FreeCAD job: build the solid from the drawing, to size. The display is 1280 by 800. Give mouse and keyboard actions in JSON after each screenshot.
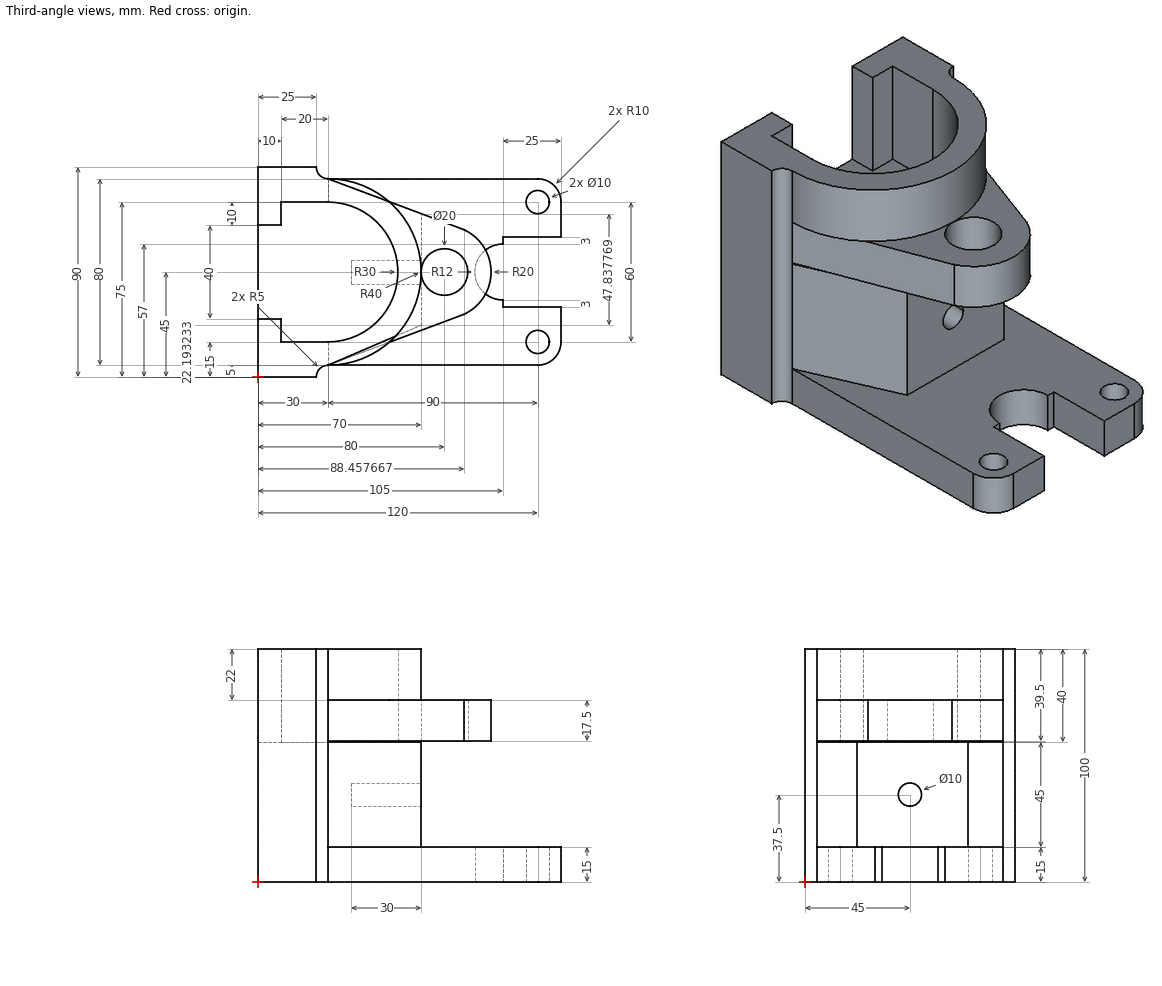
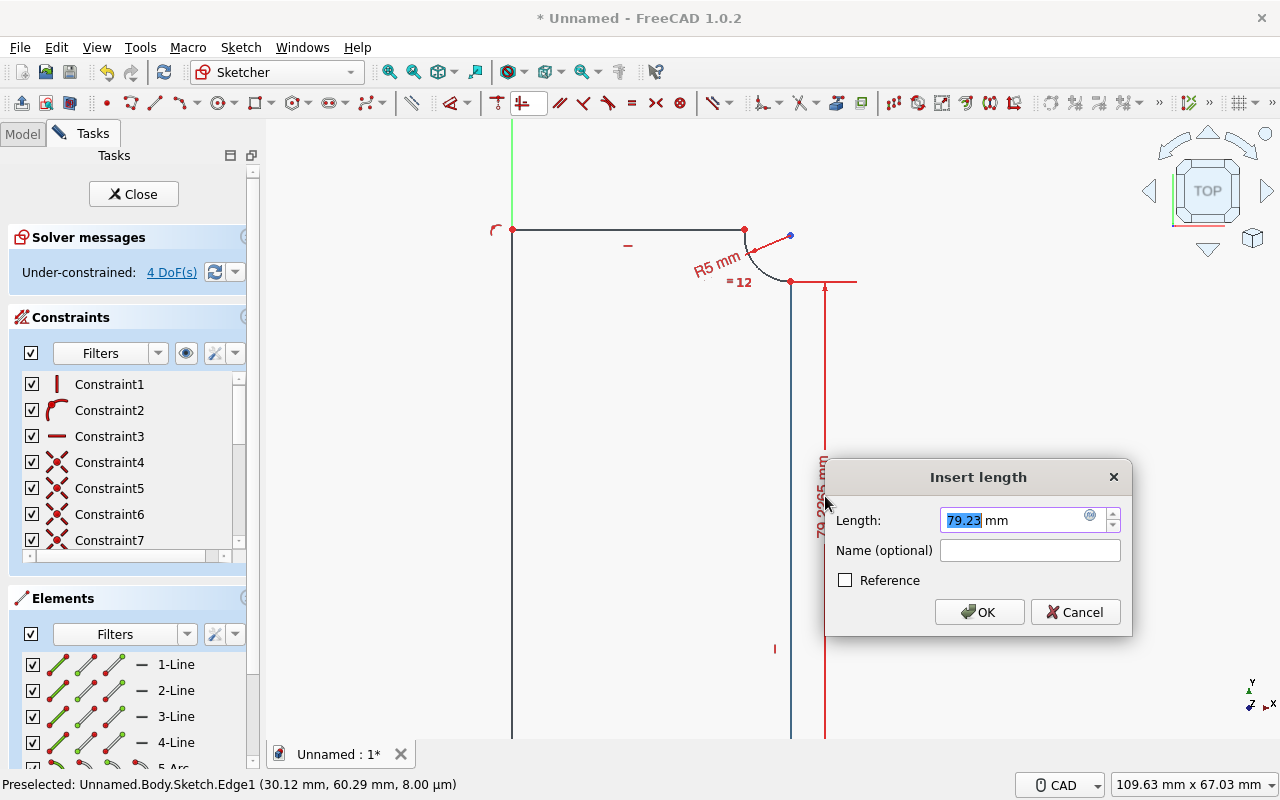
{"action": "type", "text": "80"}
{"action": "key", "text": "Return"}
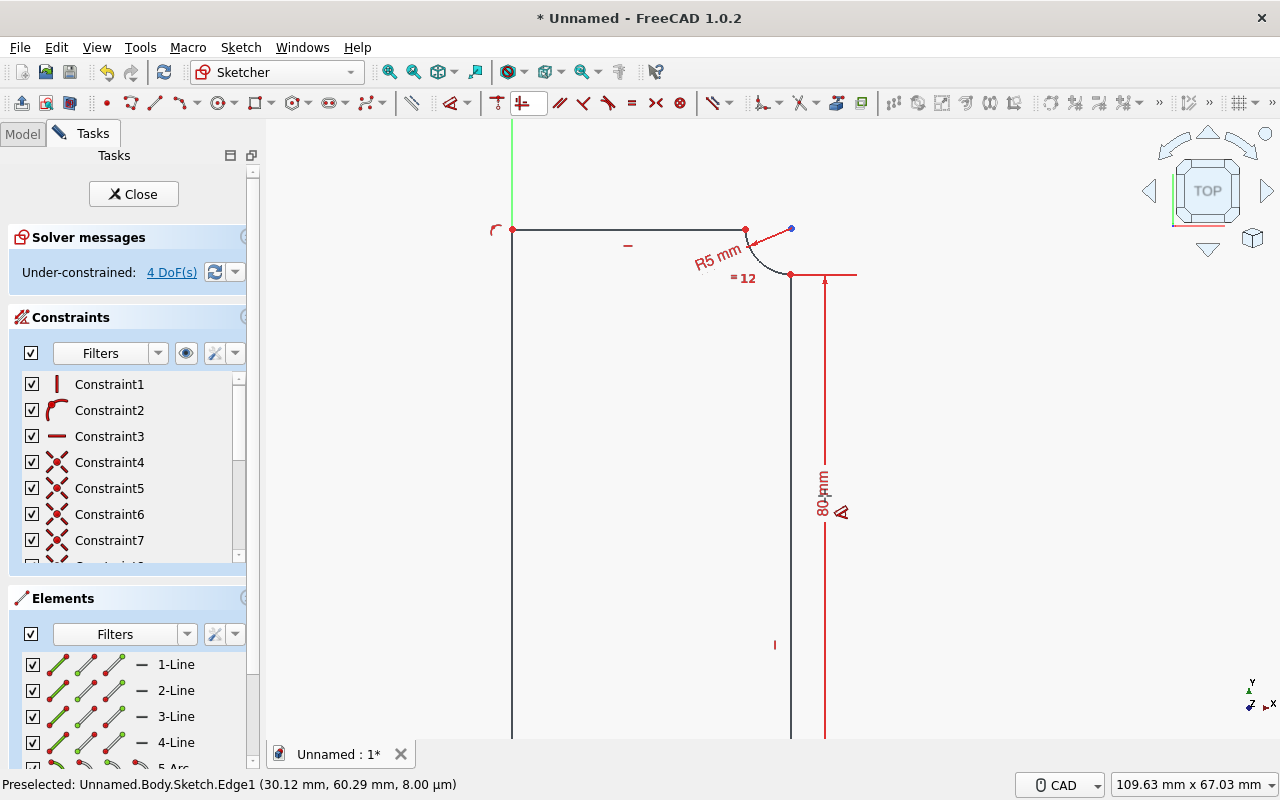
{"action": "left_click", "coordinate": [675, 230]}
{"action": "left_click", "coordinate": [629, 196]}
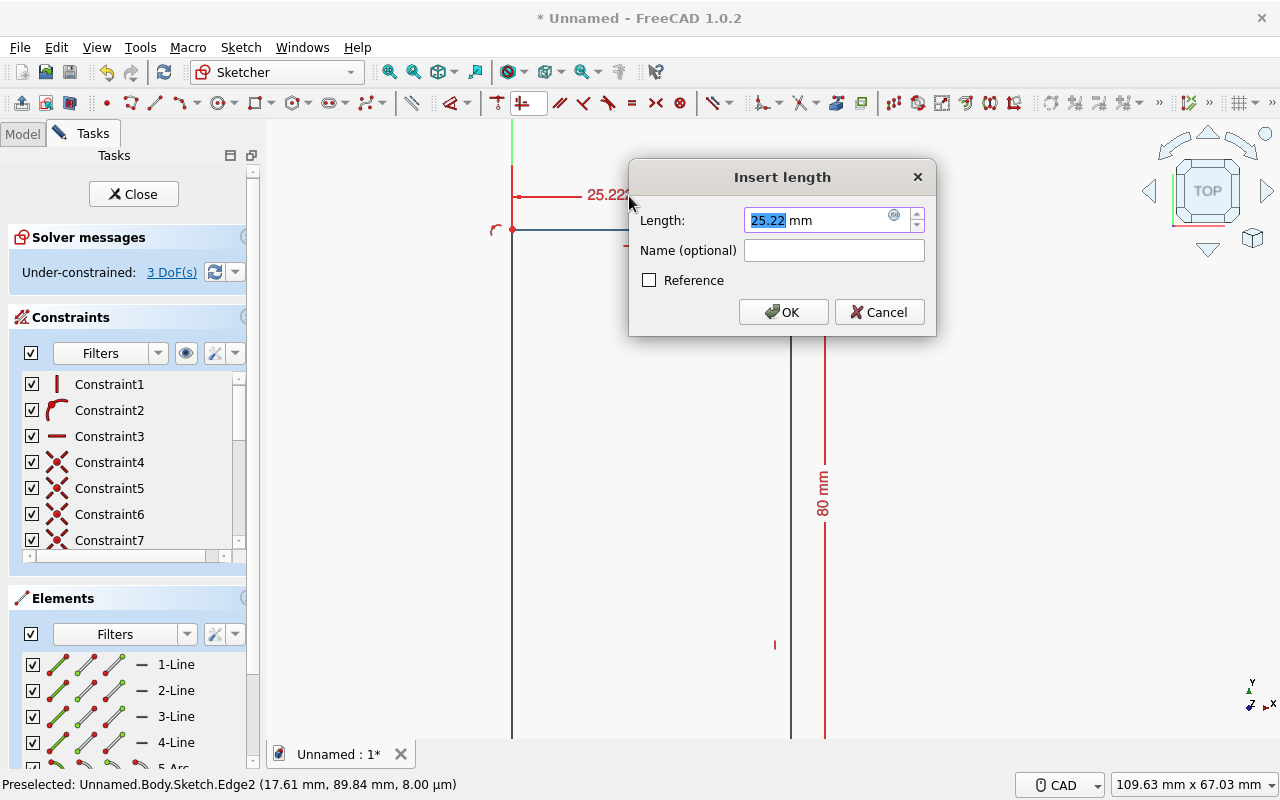
{"action": "type", "text": "25"}
{"action": "key", "text": "Return"}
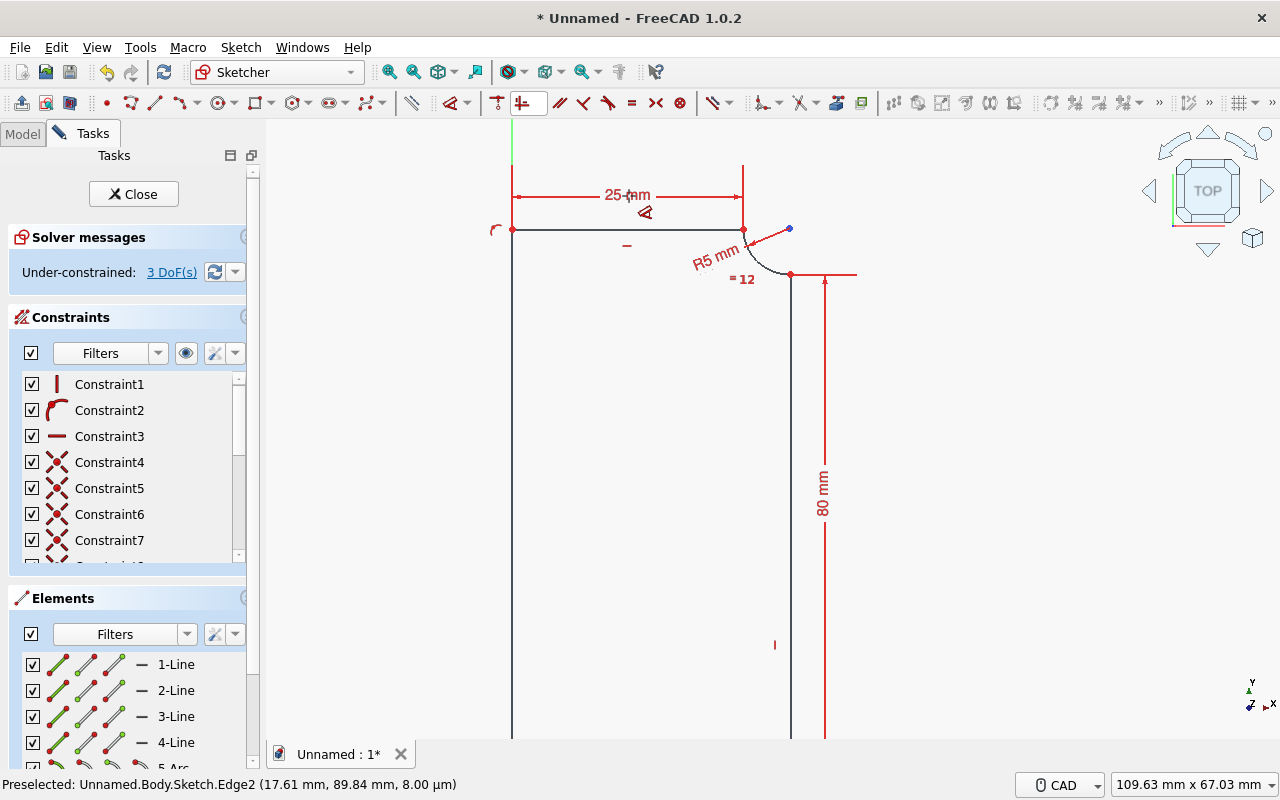
{"action": "left_click", "coordinate": [512, 479]}
{"action": "left_click", "coordinate": [478, 470]}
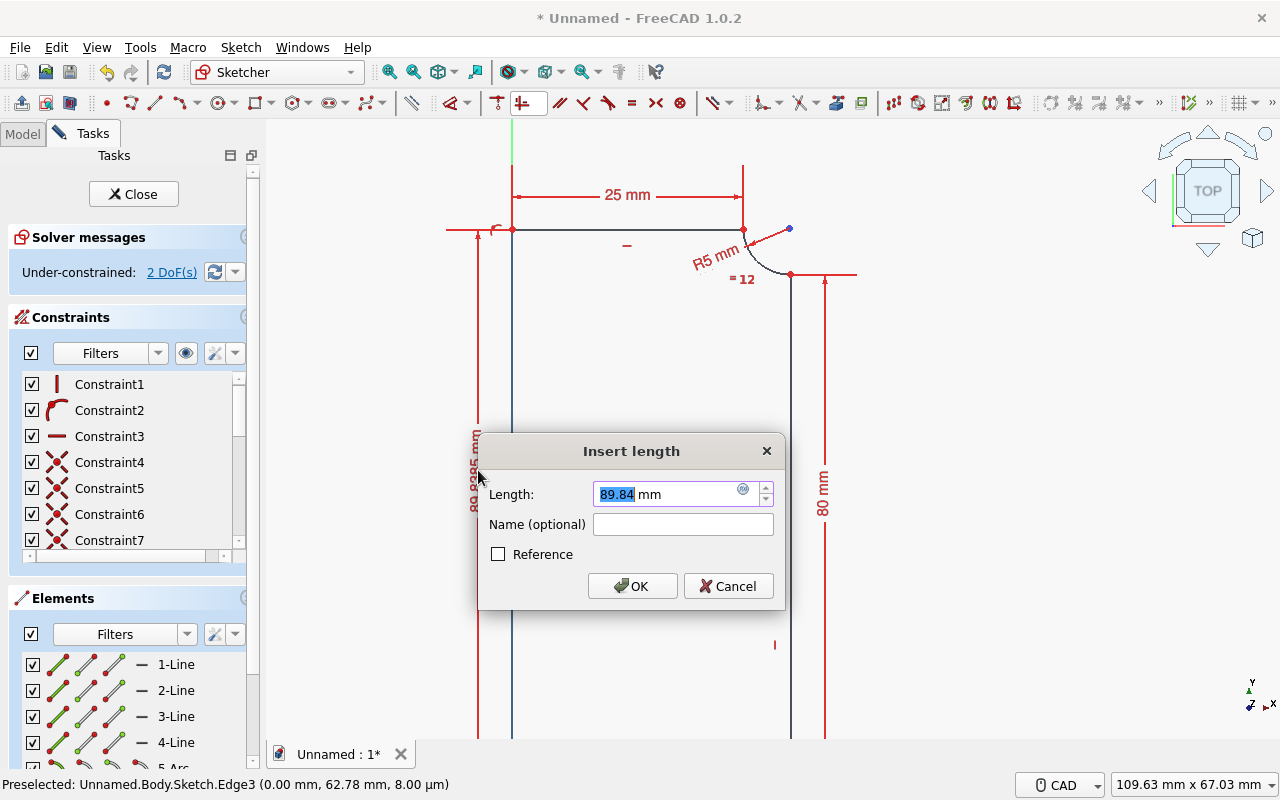
{"action": "type", "text": "90"}
{"action": "key", "text": "Return"}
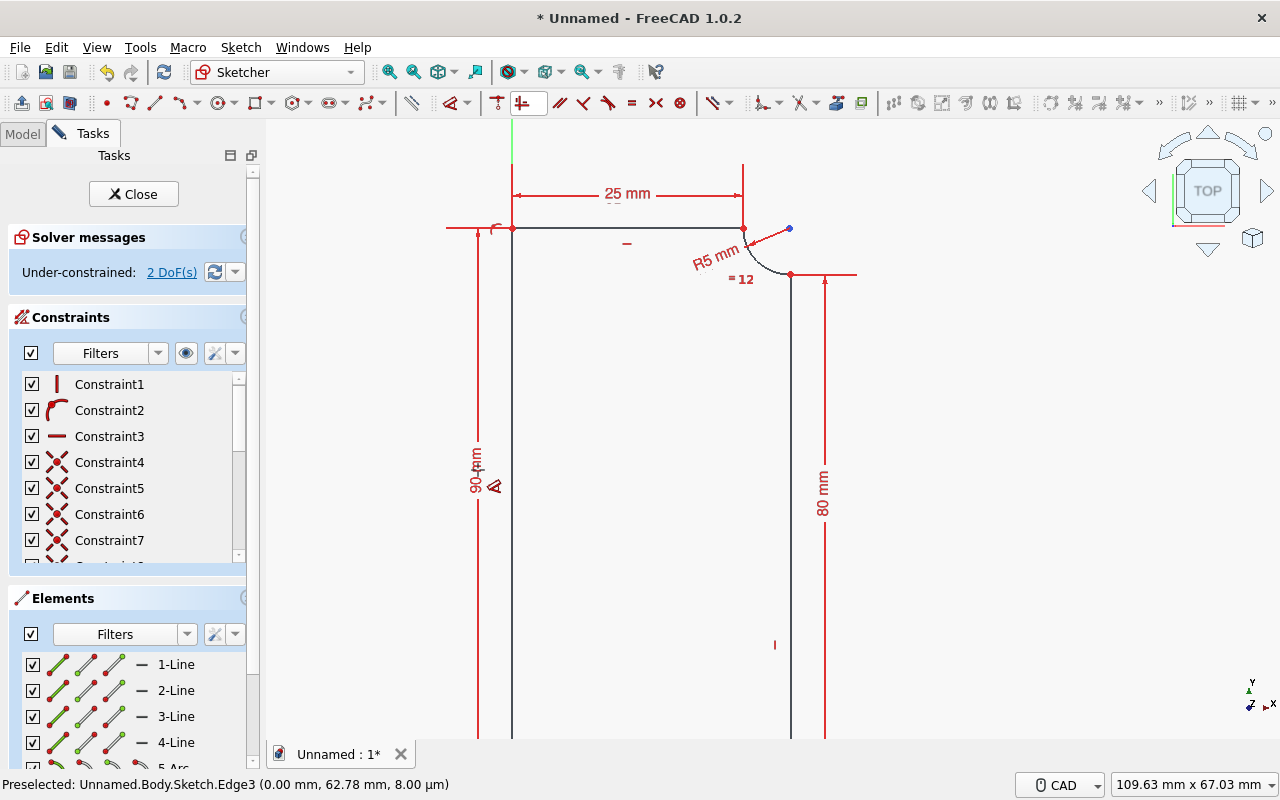
{"action": "scroll", "coordinate": [748, 253], "scroll_direction": "down", "scroll_amount": 4}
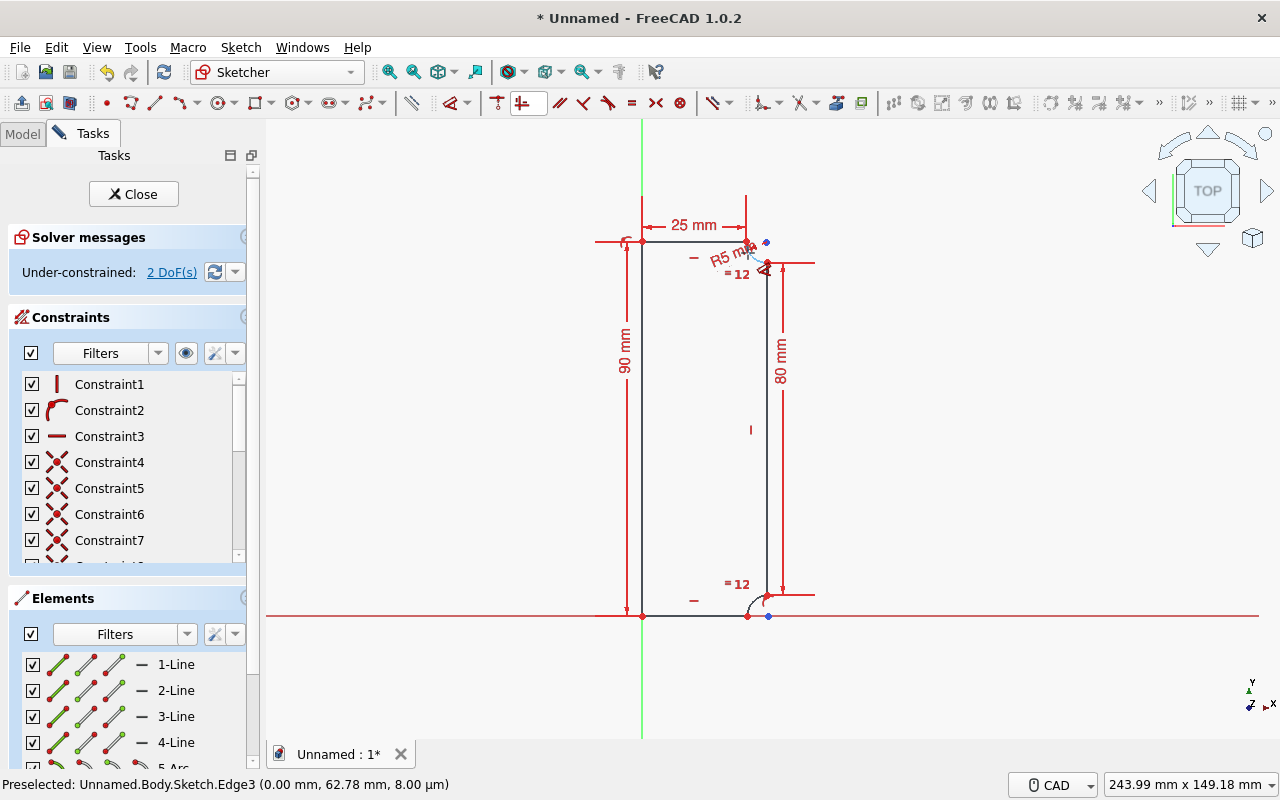
{"action": "left_click", "coordinate": [674, 616]}
{"action": "left_click", "coordinate": [695, 650]}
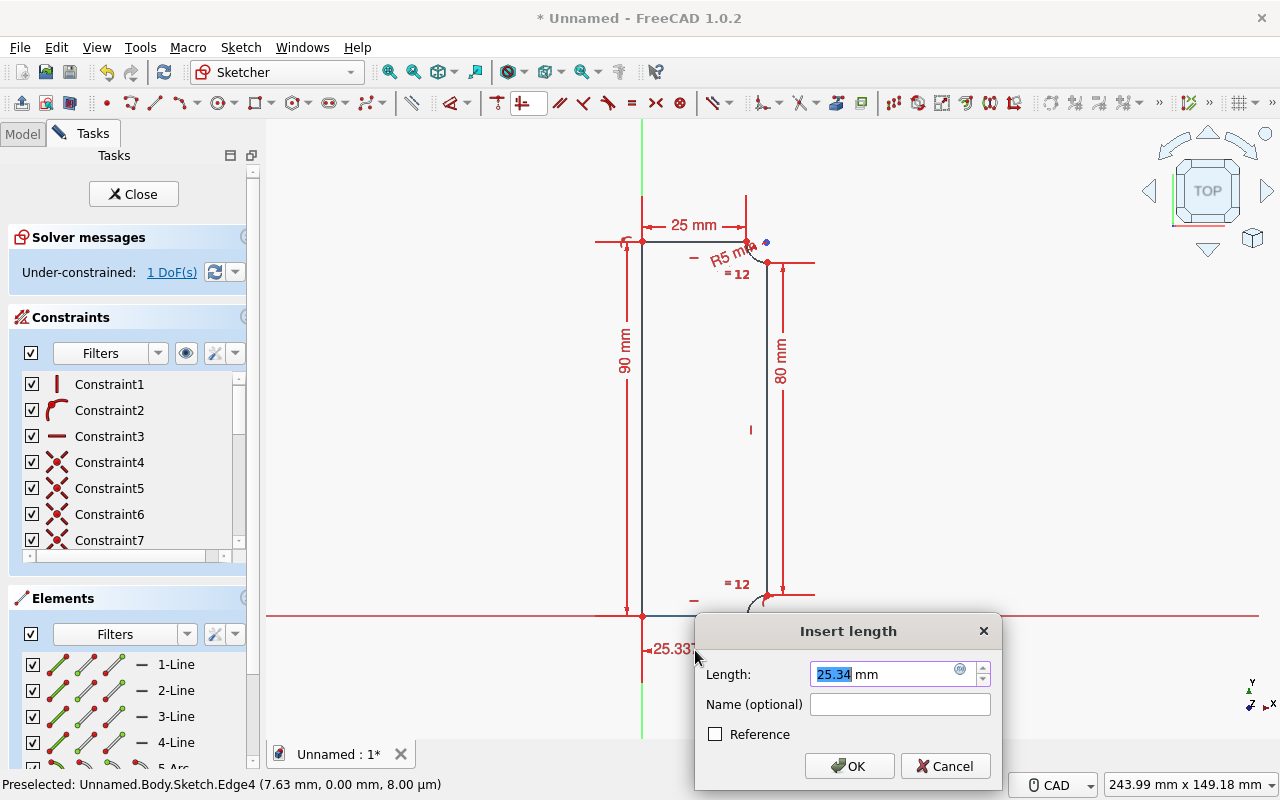
{"action": "type", "text": "25"}
{"action": "key", "text": "Return"}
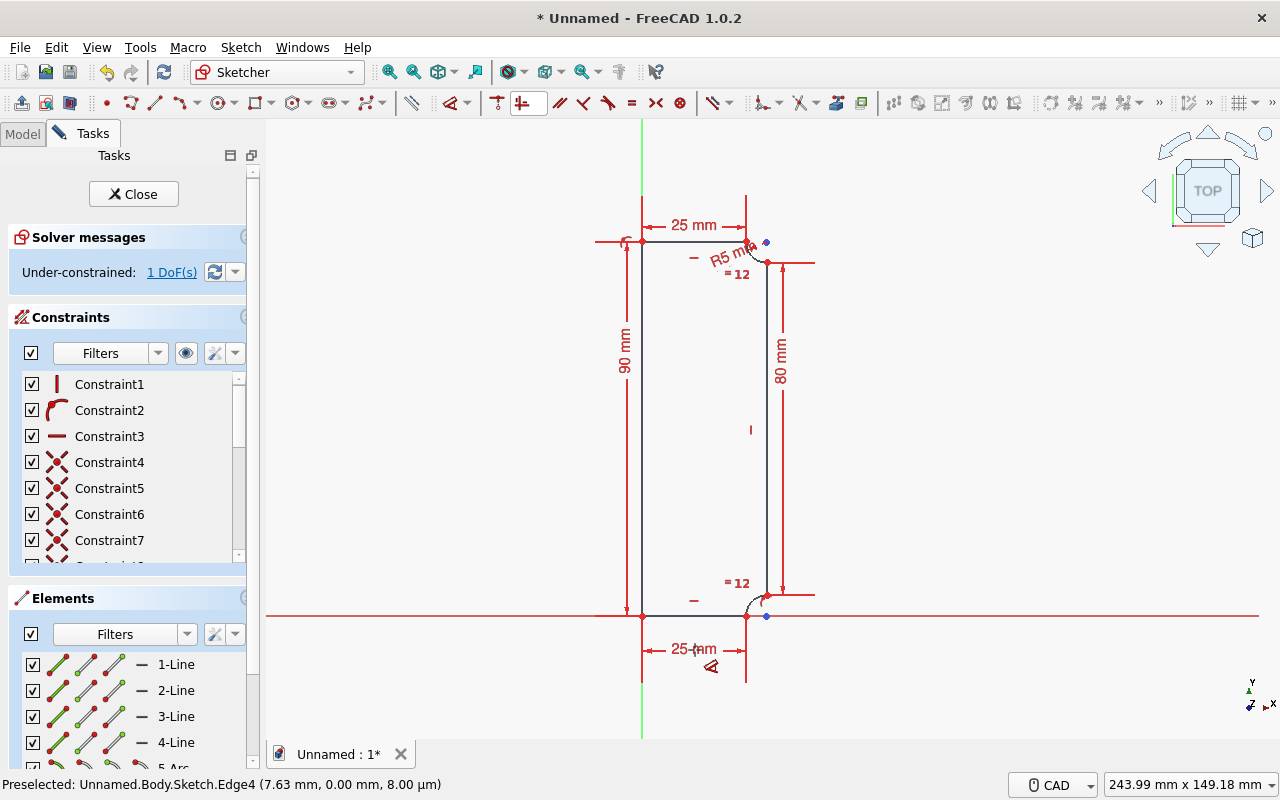
{"action": "left_click", "coordinate": [767, 595]}
{"action": "left_click", "coordinate": [705, 561]}